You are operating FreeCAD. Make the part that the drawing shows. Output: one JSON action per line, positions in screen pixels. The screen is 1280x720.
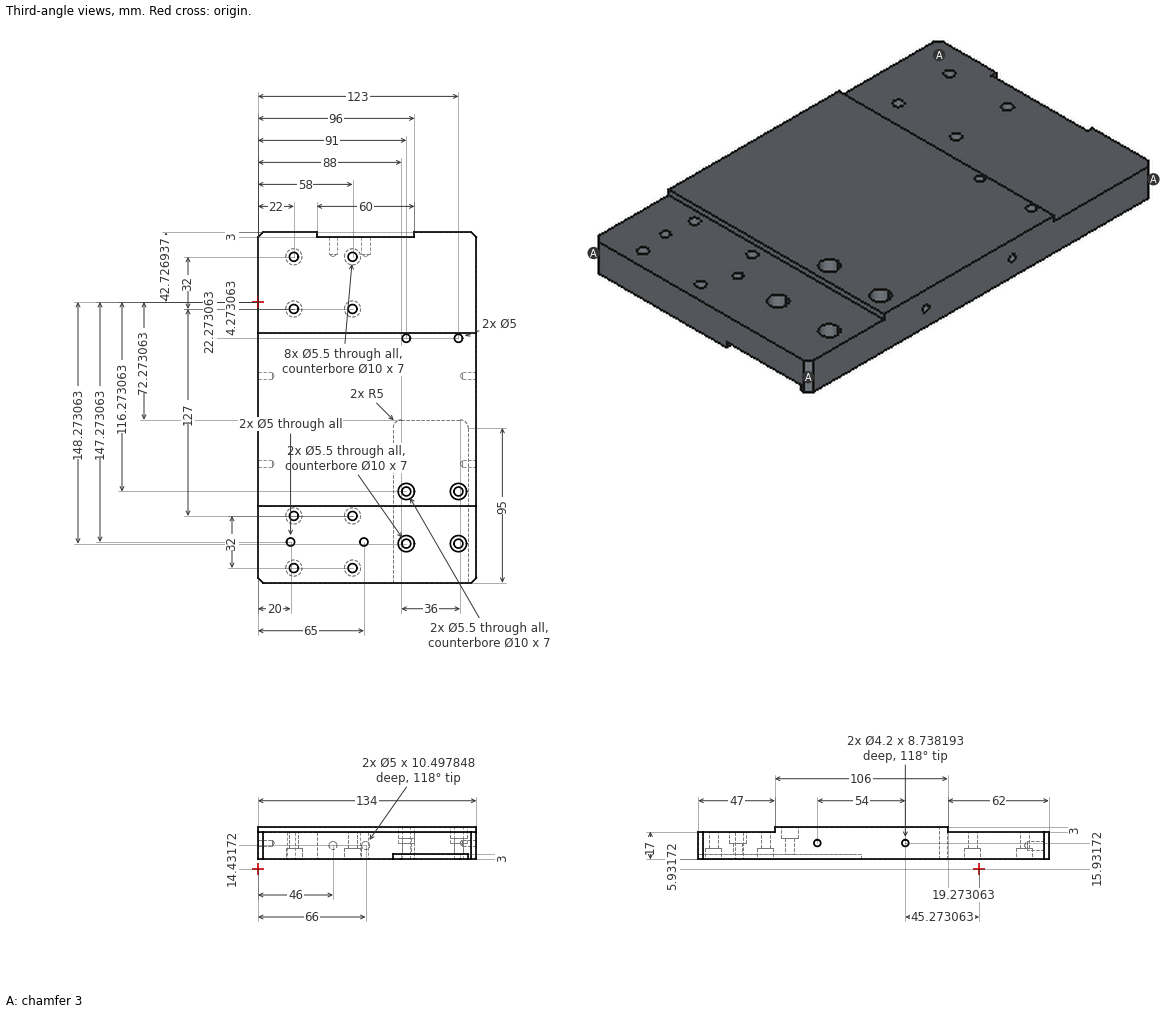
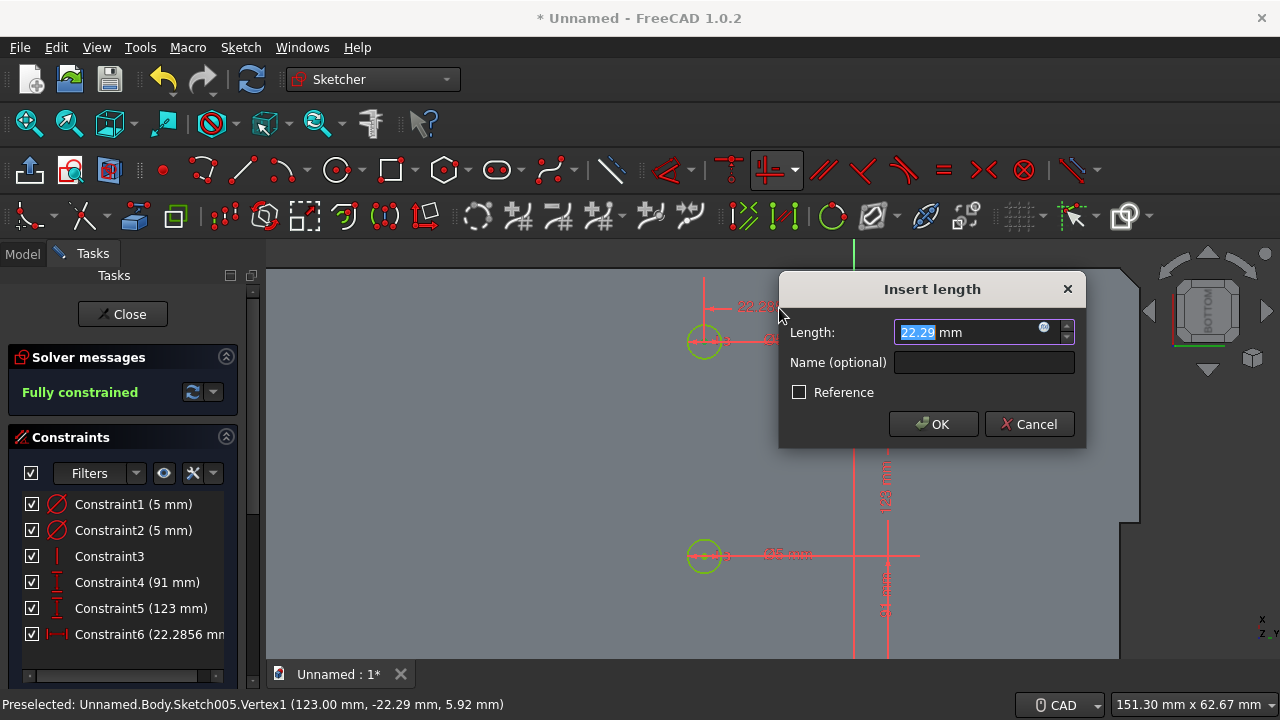
{"action": "type", "text": "22.273063"}
{"action": "key", "text": "Return"}
{"action": "key", "text": "Escape"}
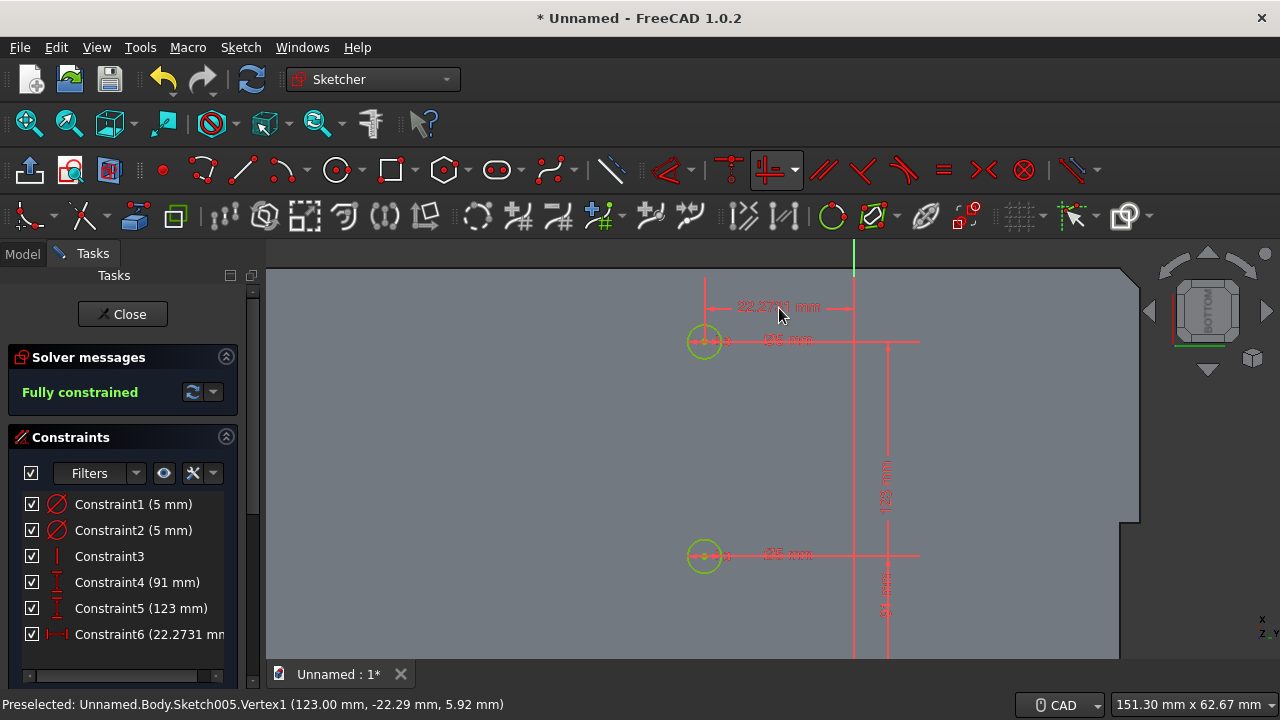
{"action": "left_click", "coordinate": [123, 314]}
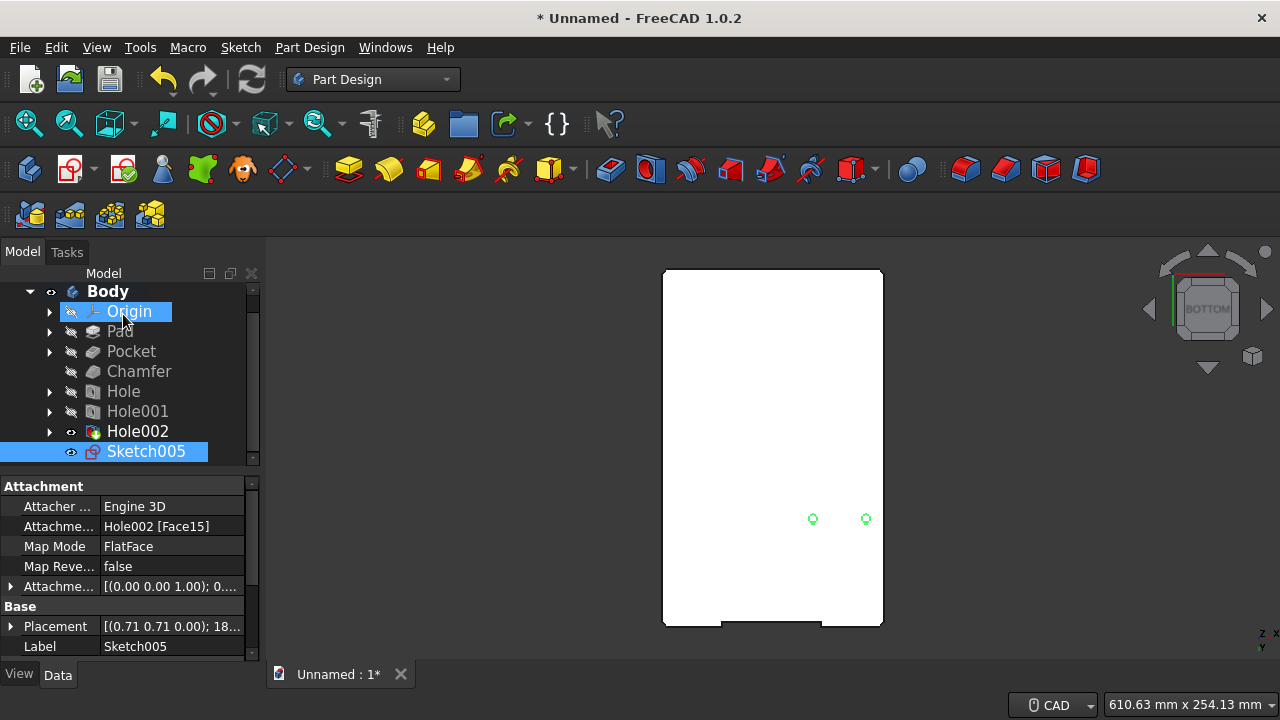
{"action": "left_click", "coordinate": [612, 170]}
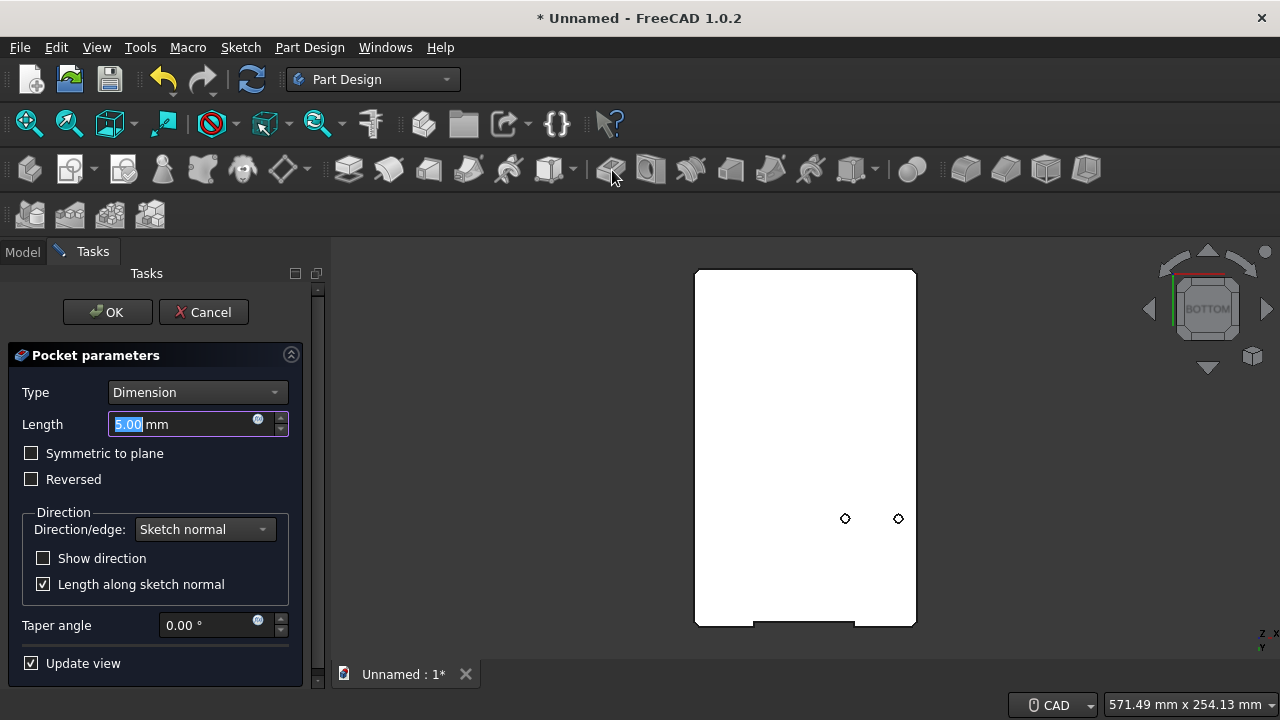
{"action": "left_click", "coordinate": [198, 392]}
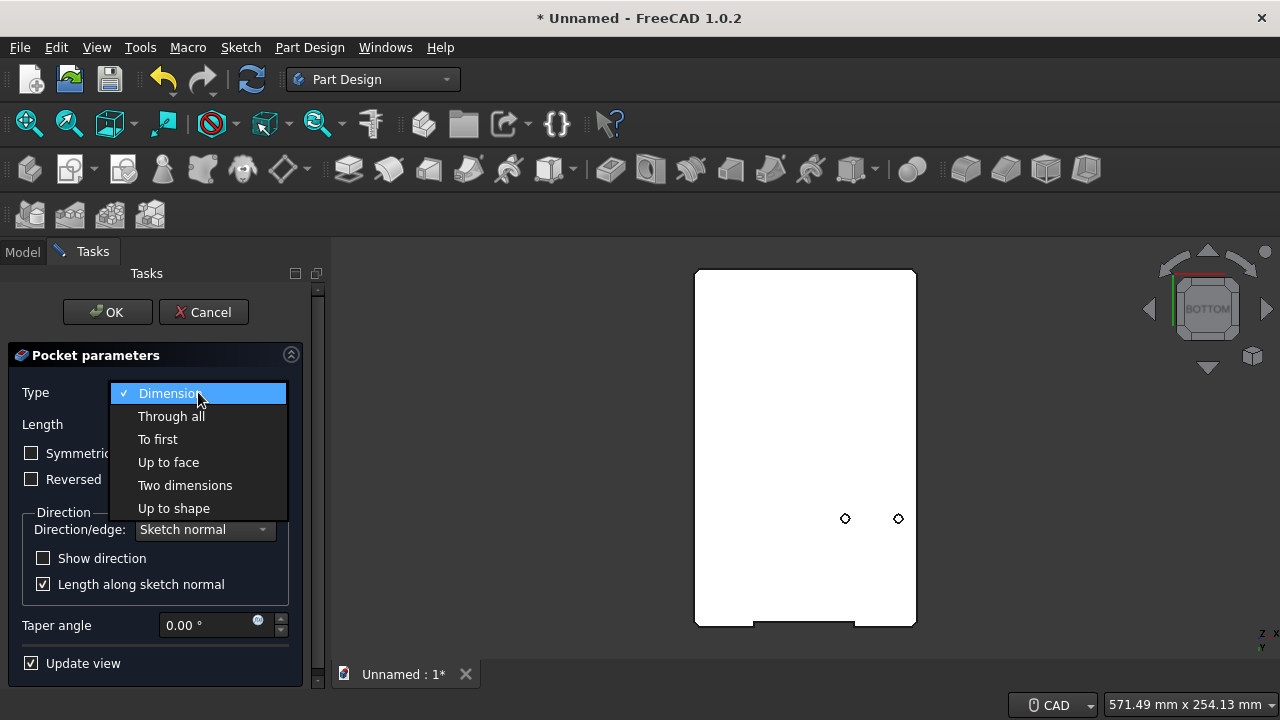
{"action": "left_click", "coordinate": [198, 416]}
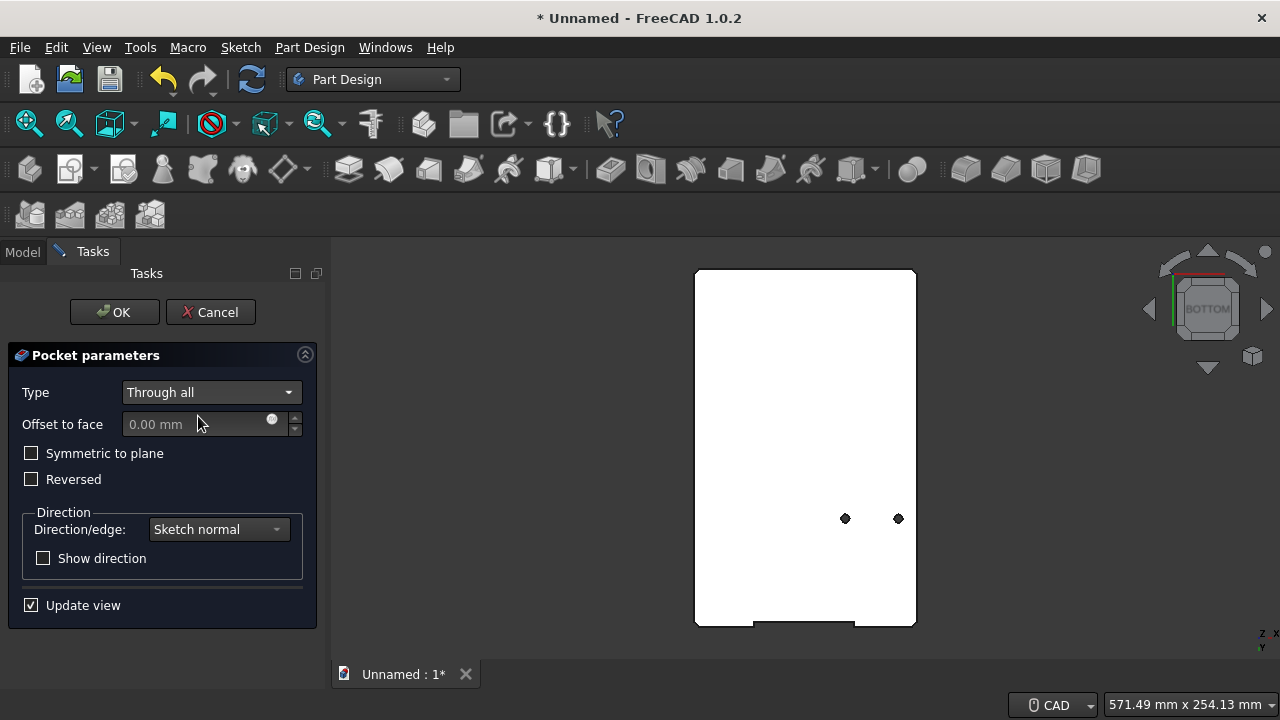
{"action": "left_click", "coordinate": [115, 312]}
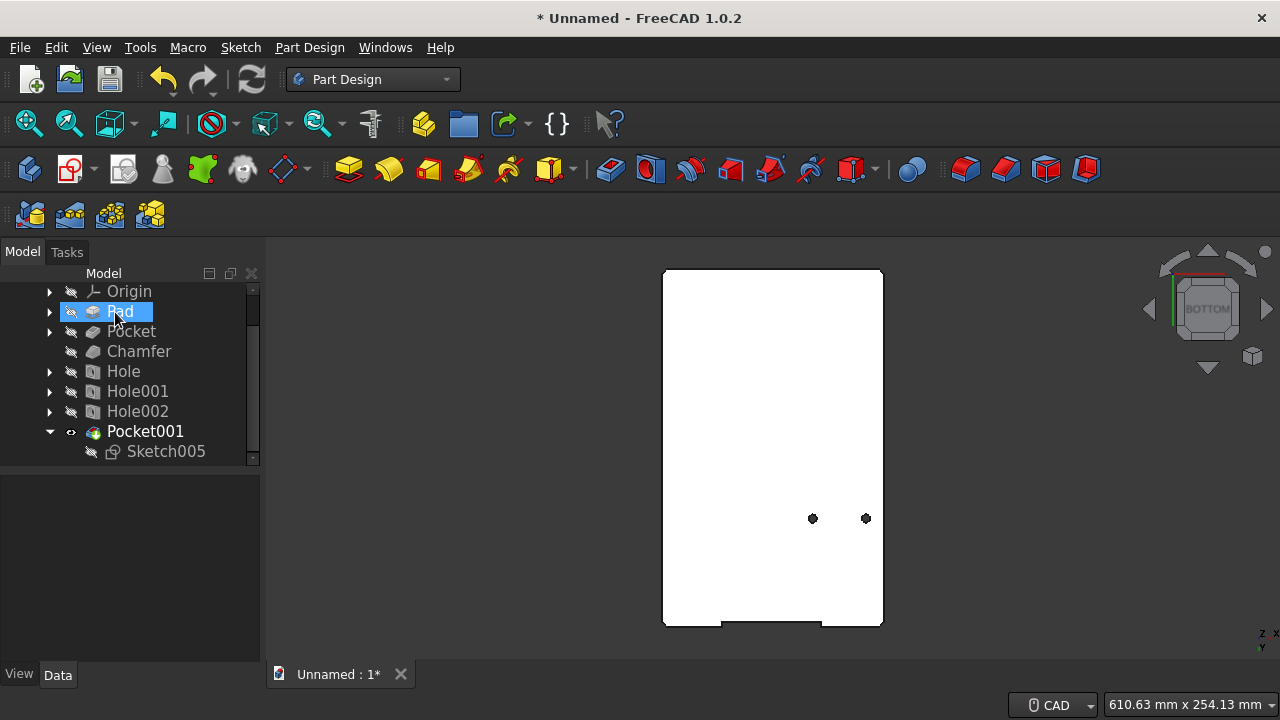
{"action": "left_click", "coordinate": [773, 396]}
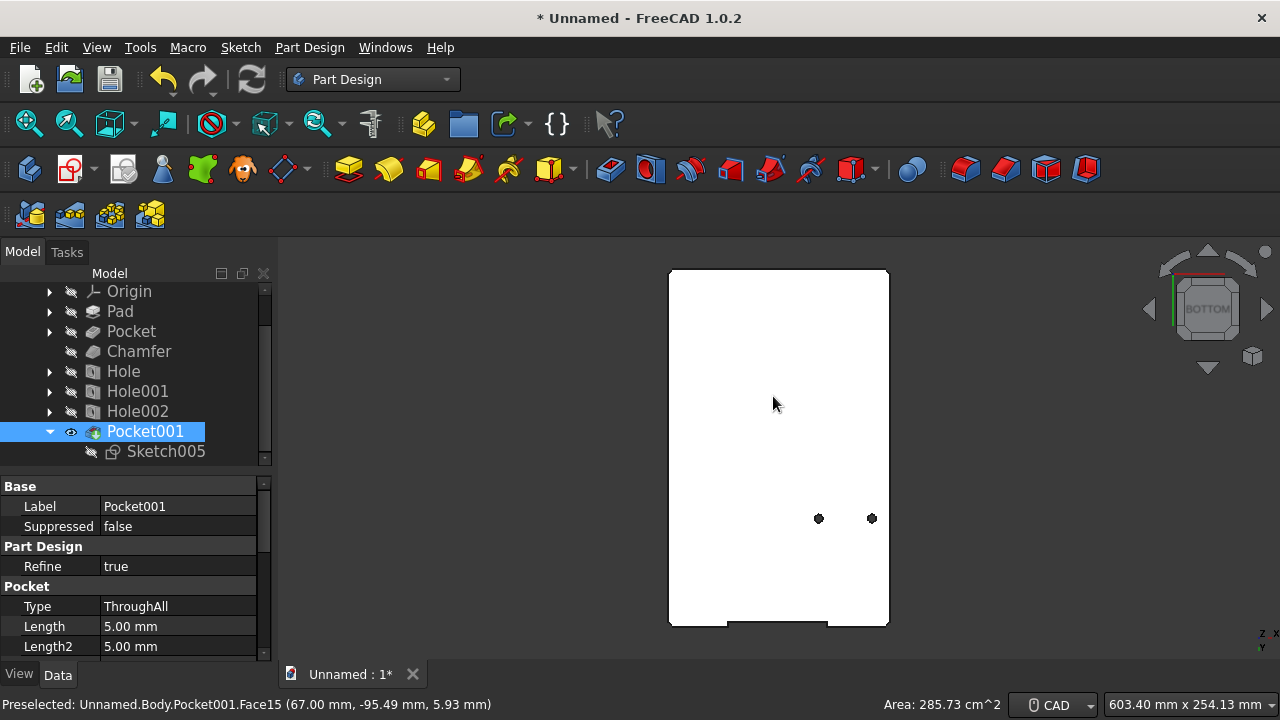
{"action": "left_click", "coordinate": [70, 170]}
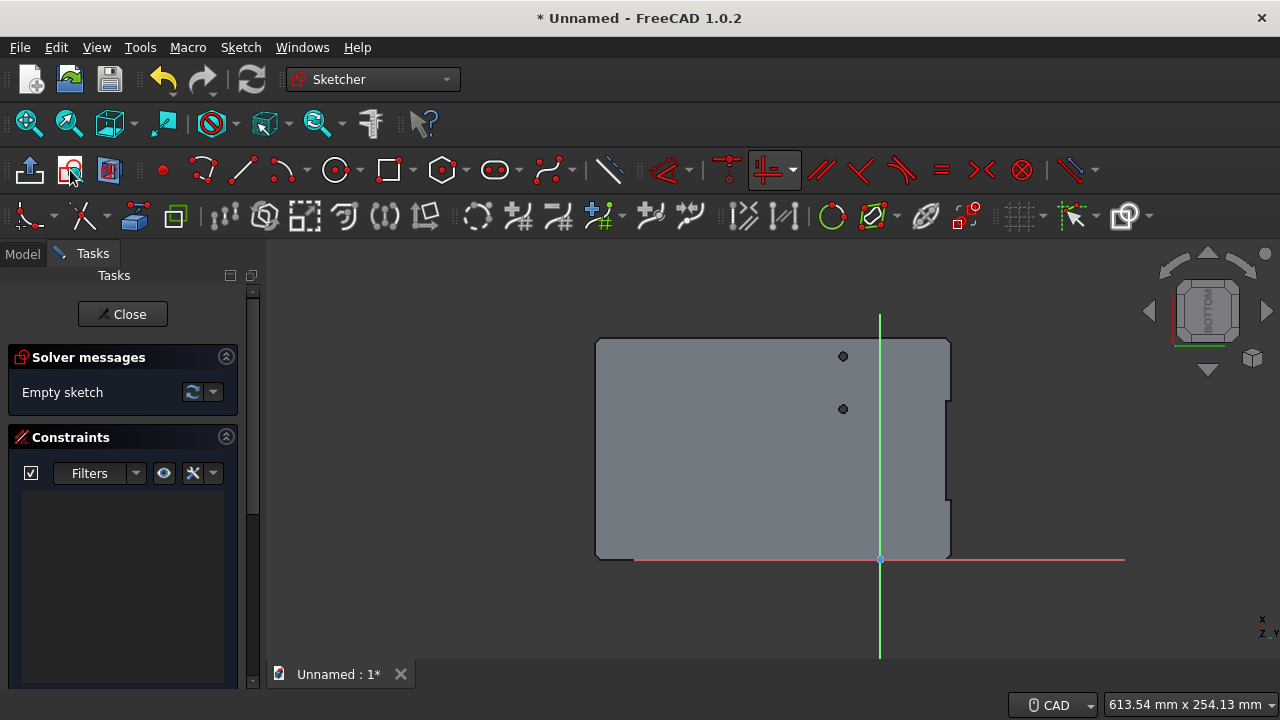
{"action": "scroll", "coordinate": [845, 583], "scroll_direction": "up", "scroll_amount": 3}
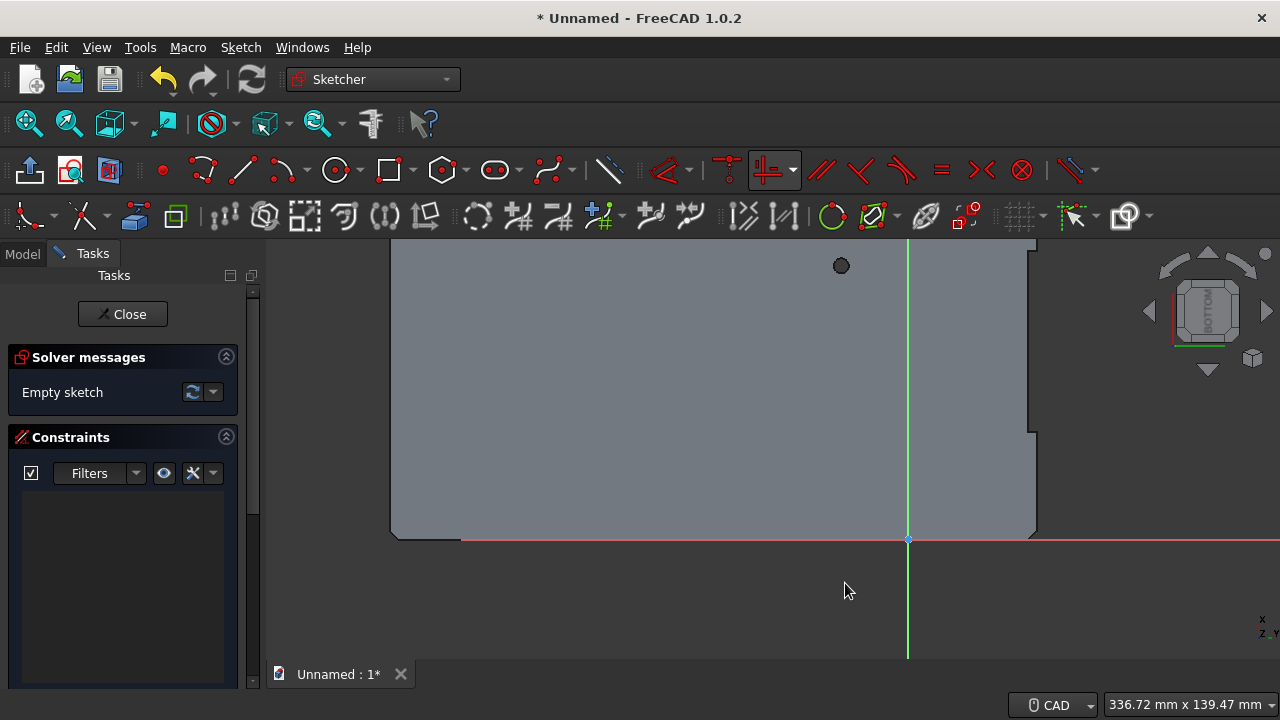
{"action": "left_click", "coordinate": [336, 170]}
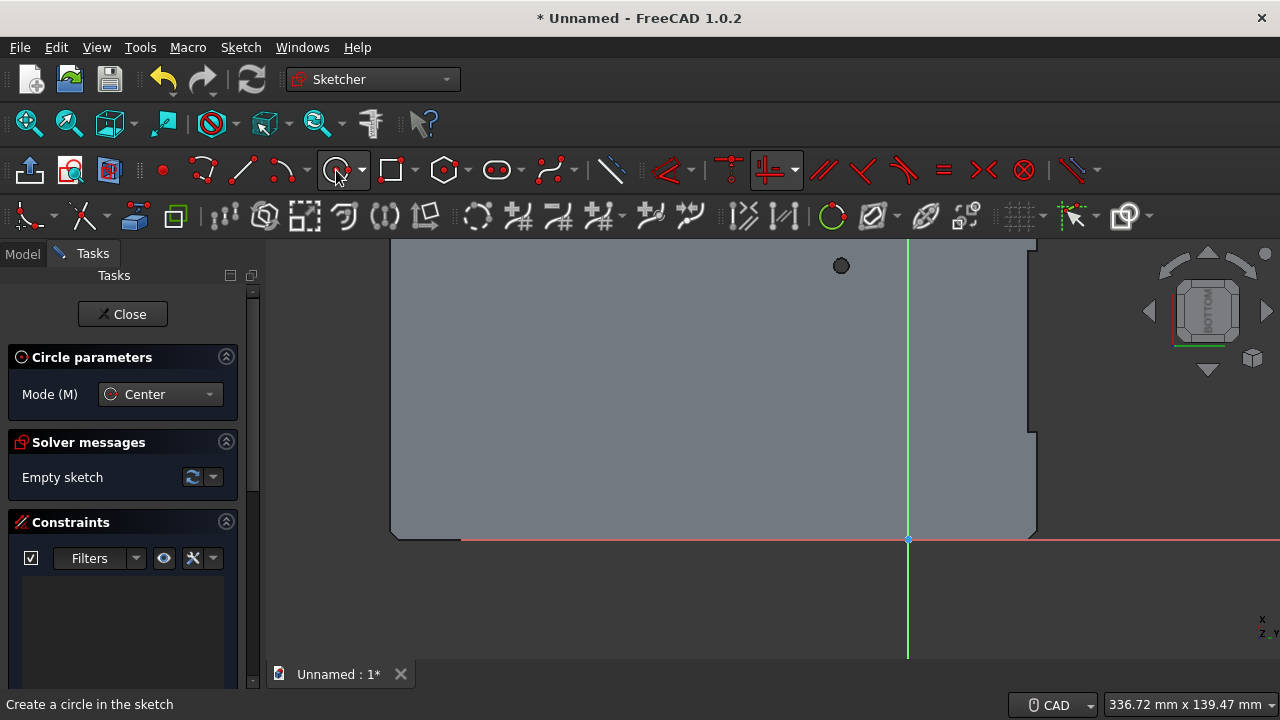
{"action": "scroll", "coordinate": [992, 365], "scroll_direction": "up", "scroll_amount": 6}